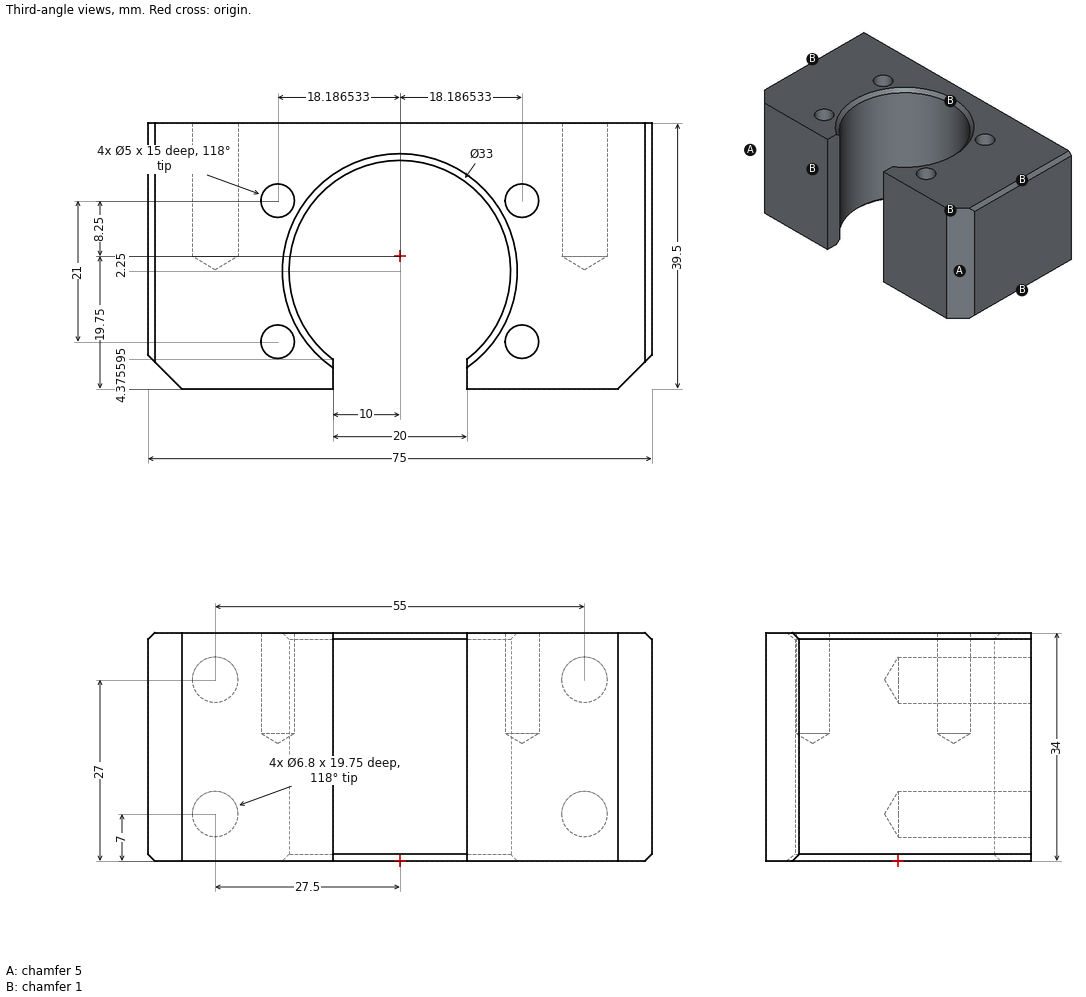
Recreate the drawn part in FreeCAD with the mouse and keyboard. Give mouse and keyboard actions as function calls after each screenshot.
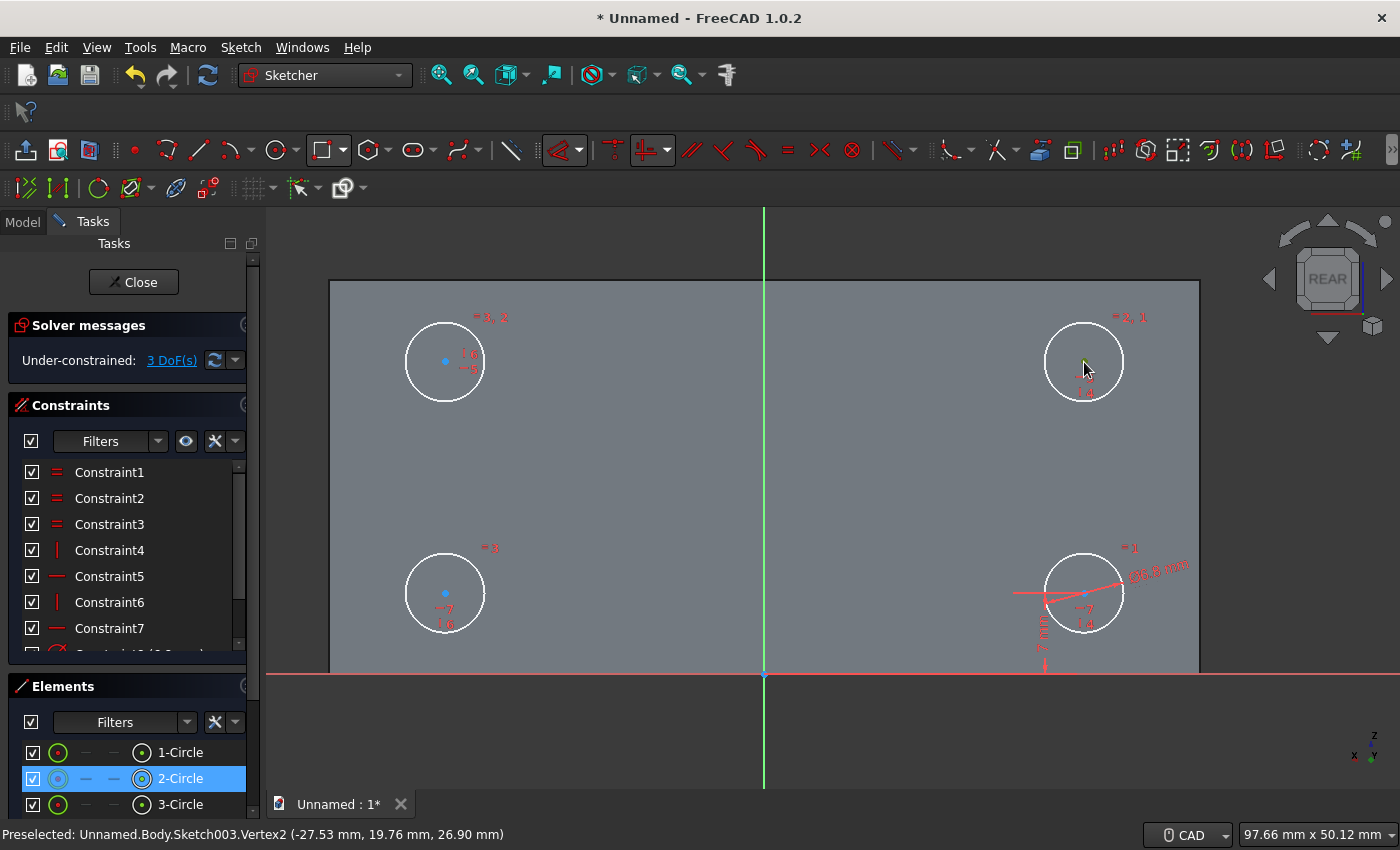
key(i)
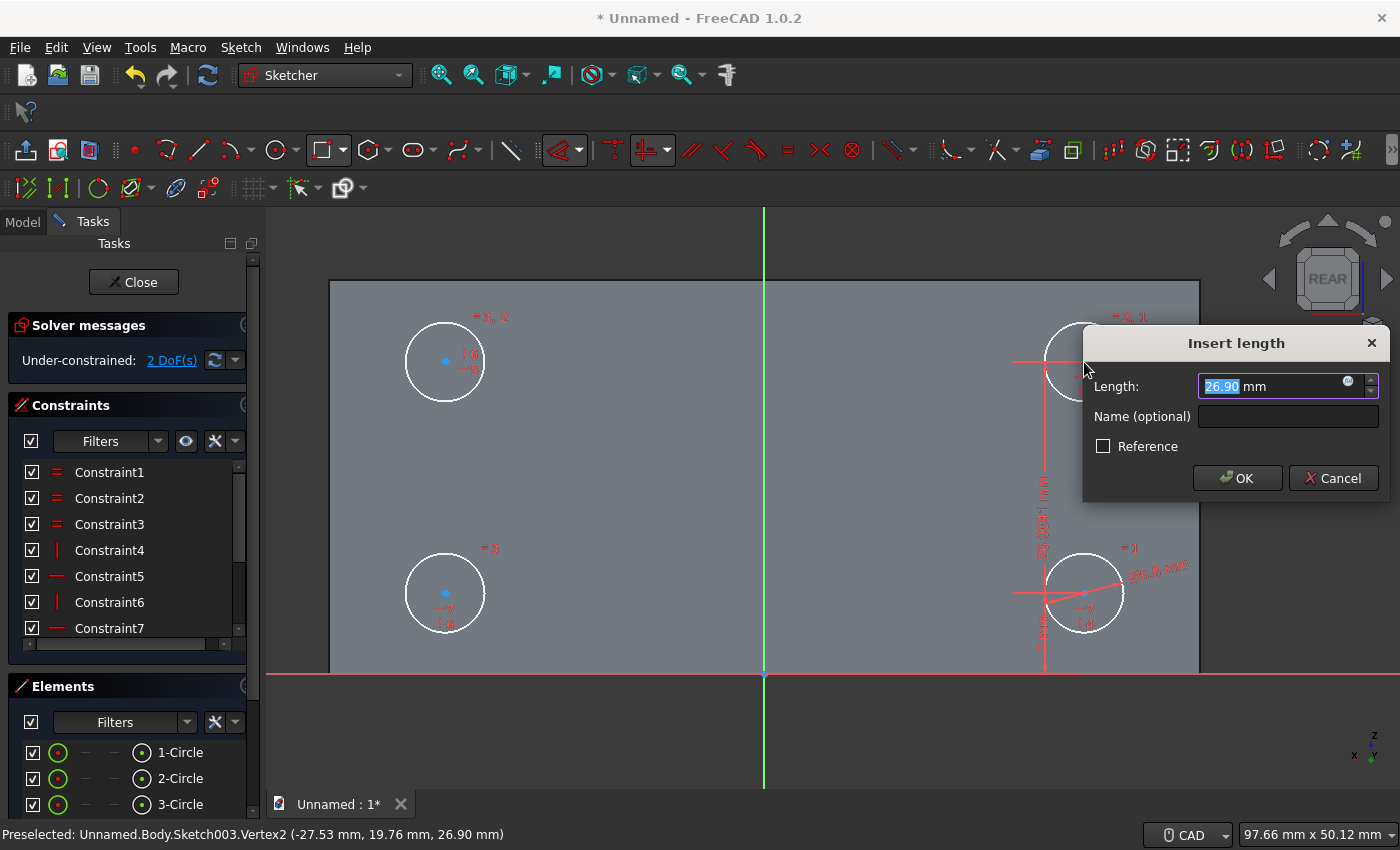
text(27)
key(Return)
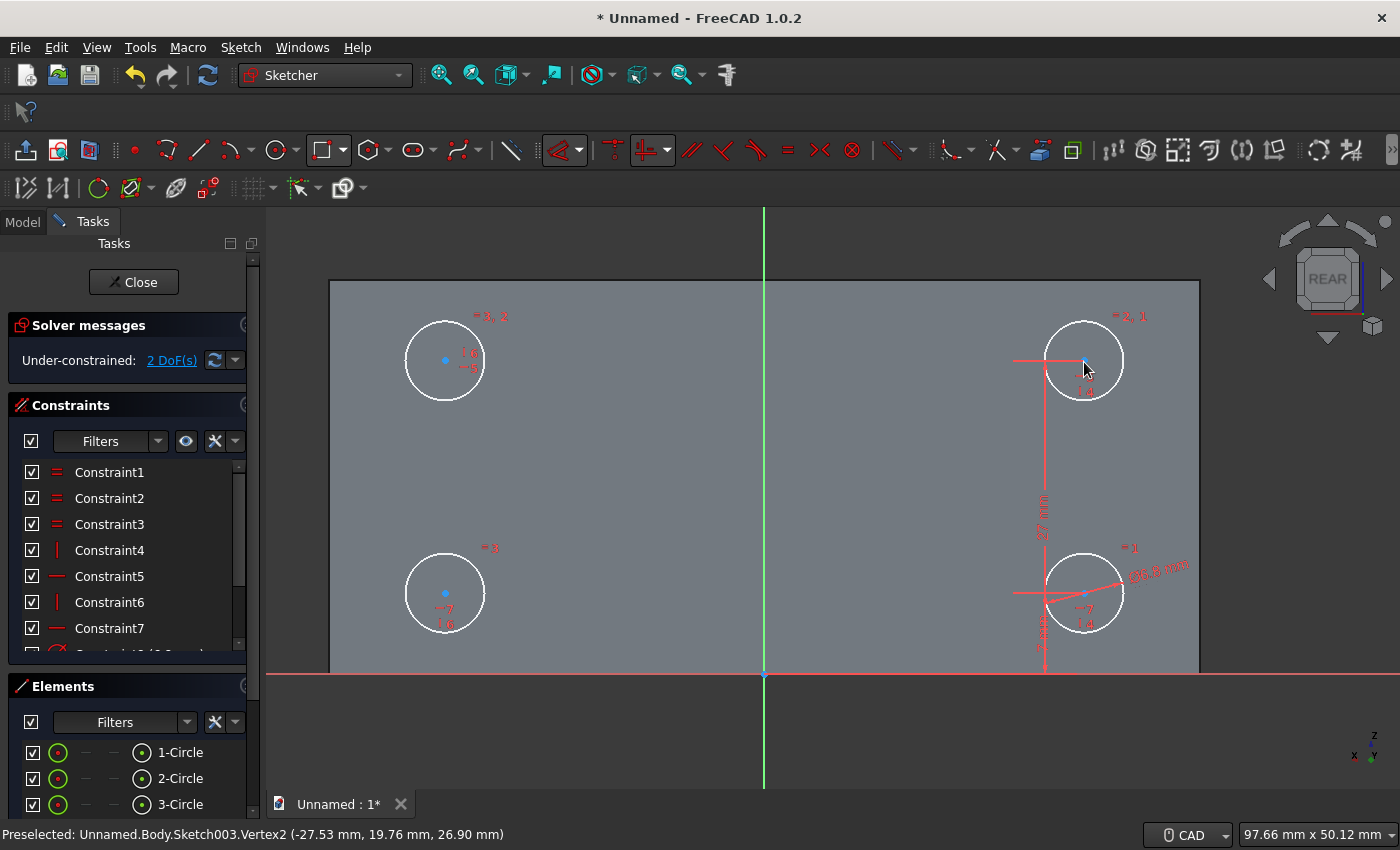
click(1084, 361)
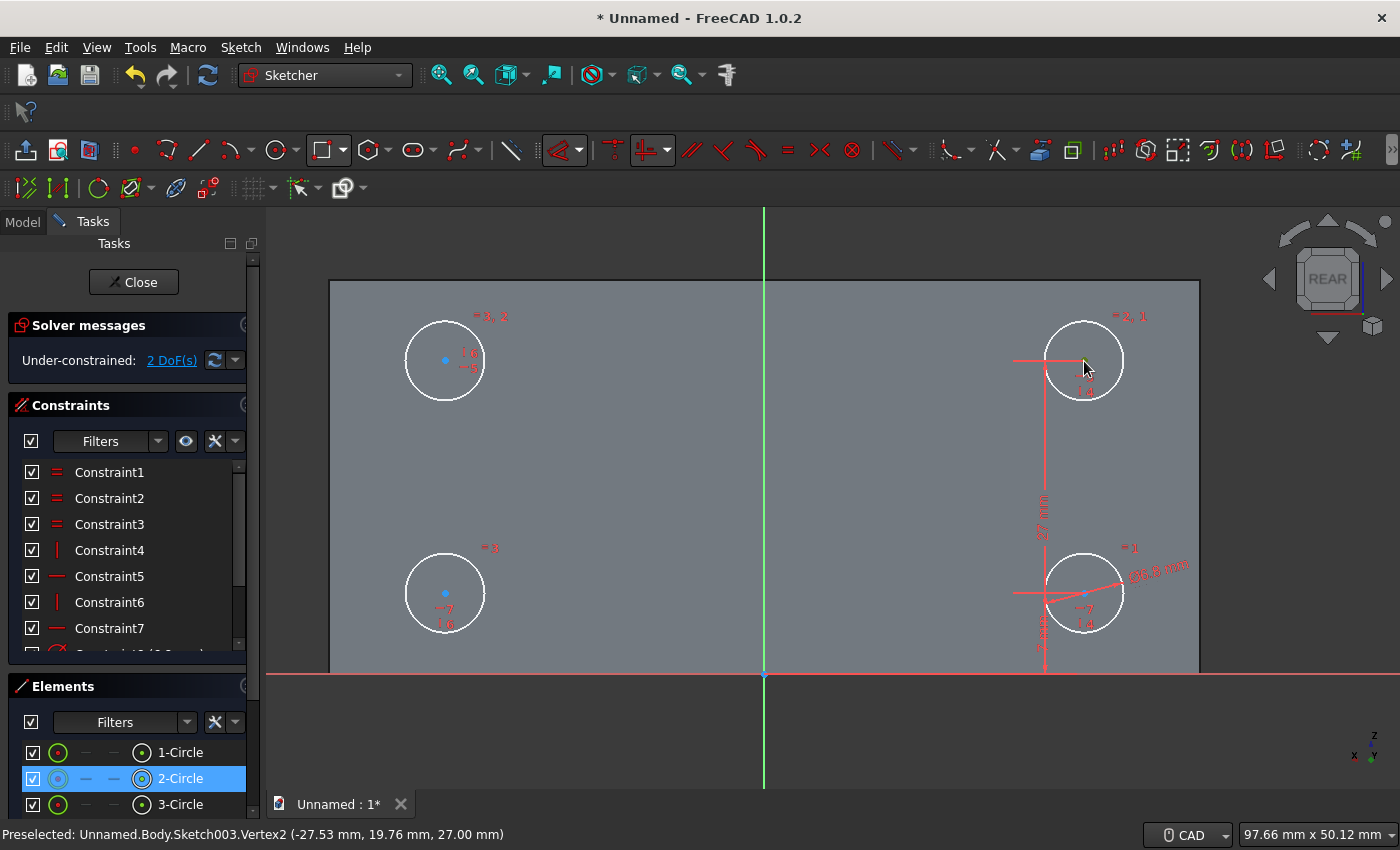
click(445, 361)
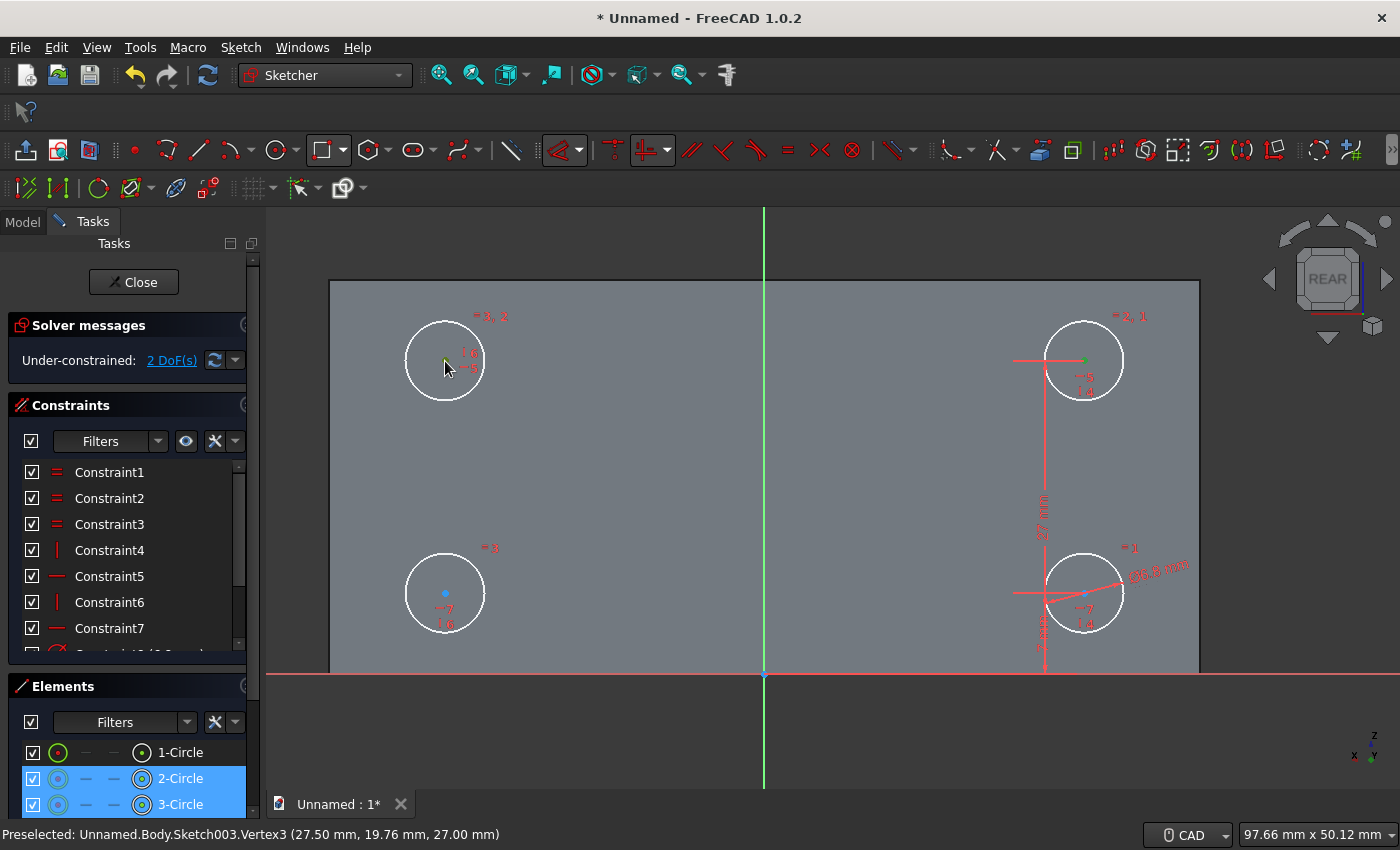
key(l)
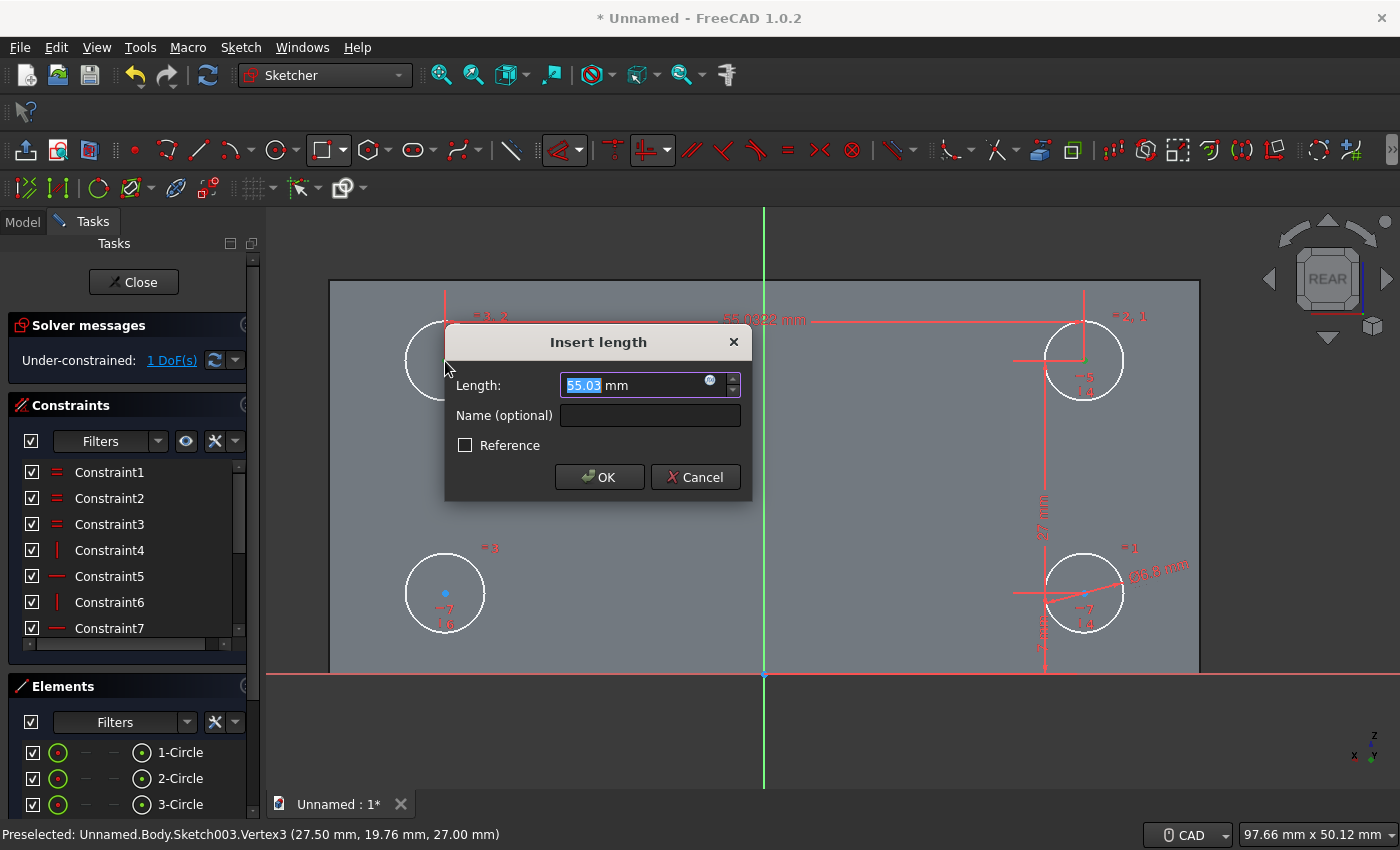
text(55)
key(Return)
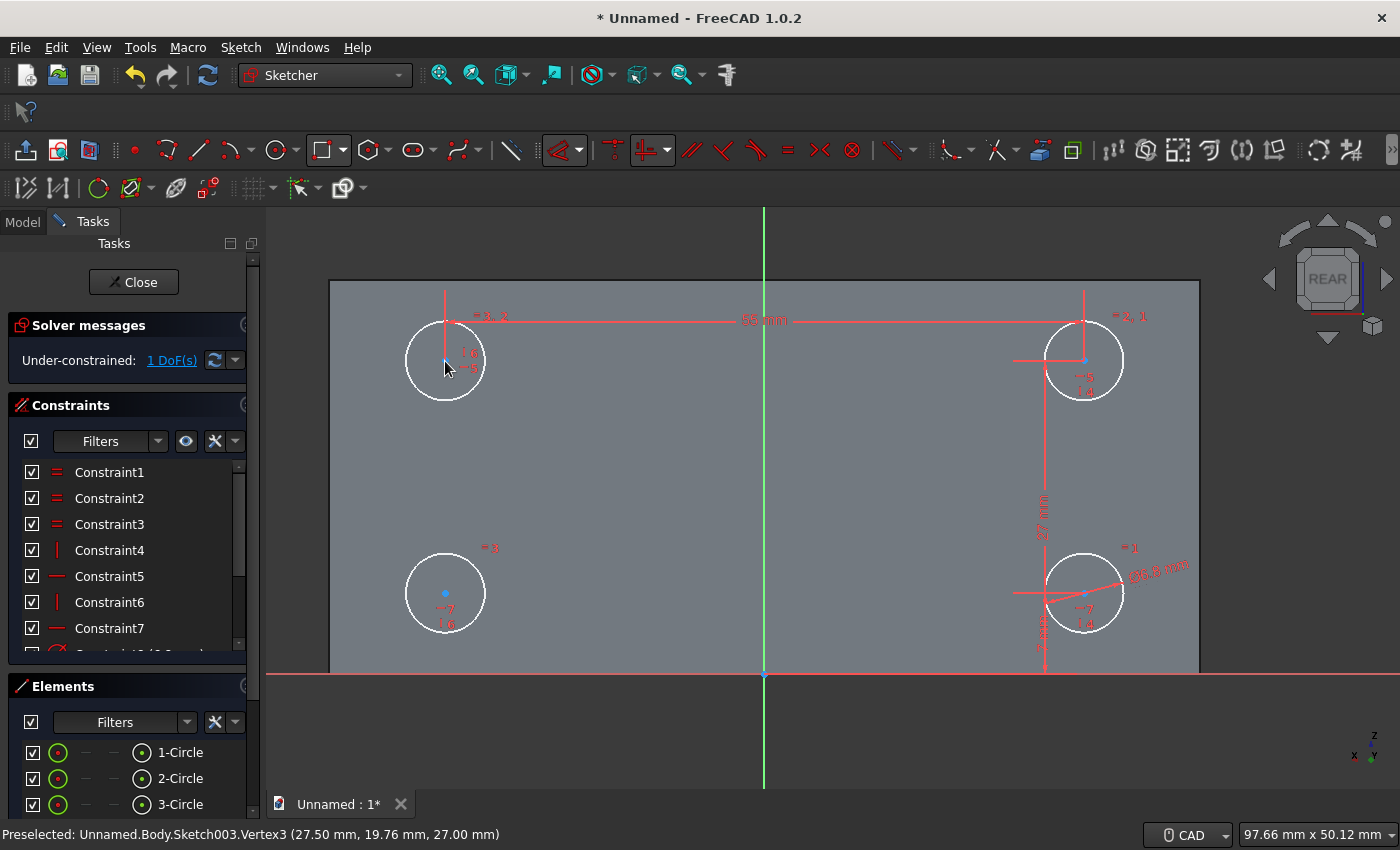
click(1084, 593)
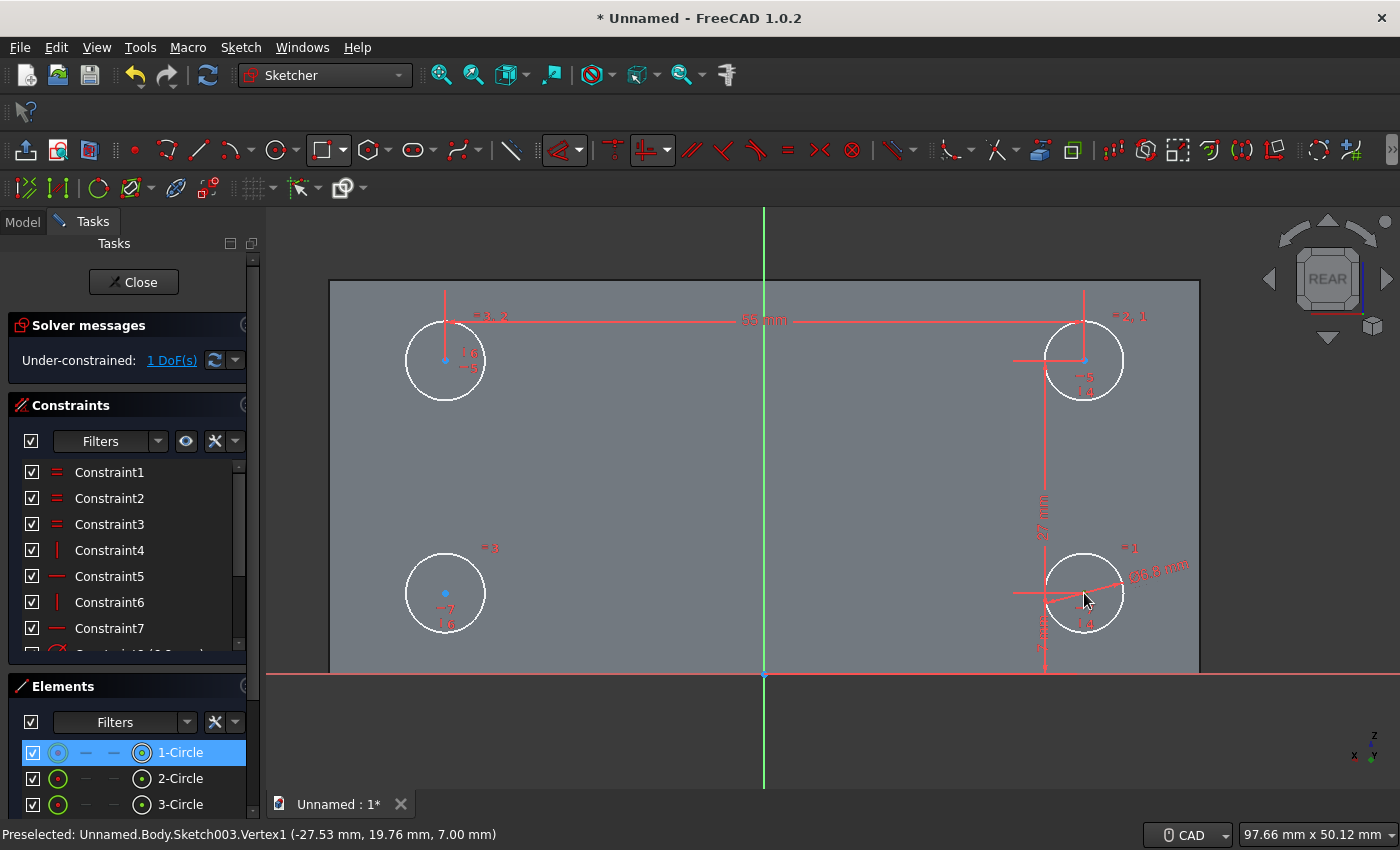
click(582, 150)